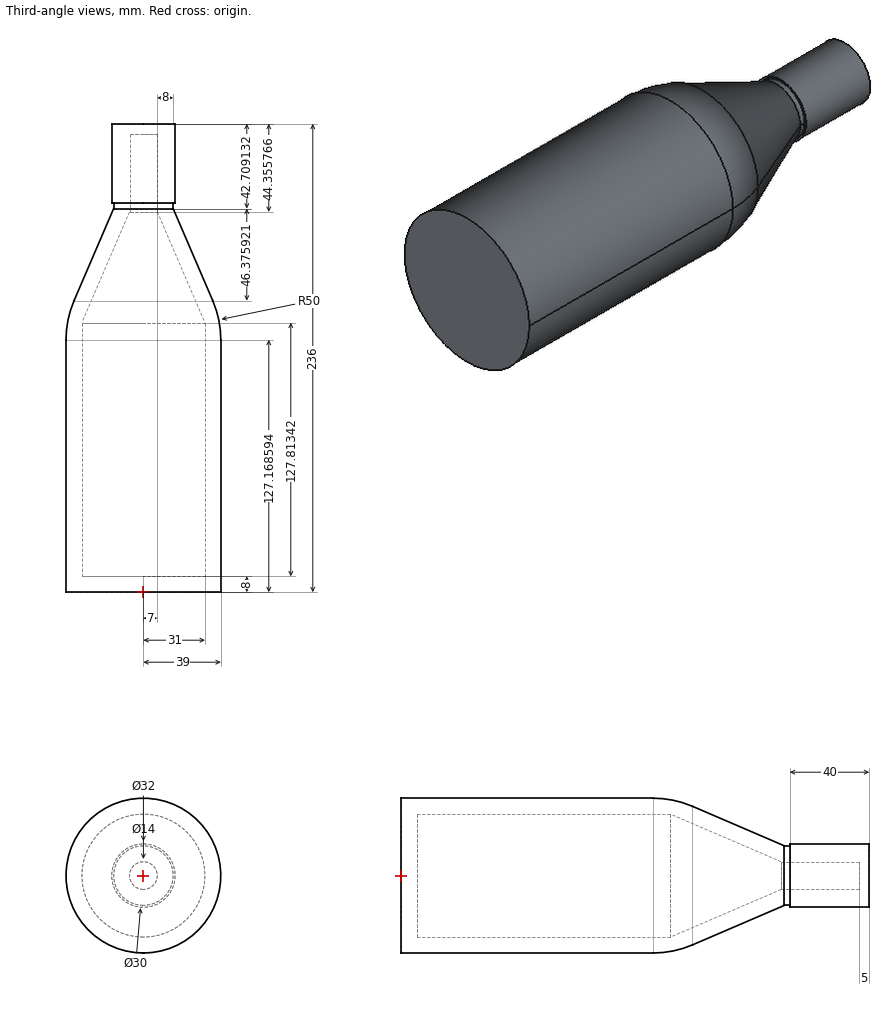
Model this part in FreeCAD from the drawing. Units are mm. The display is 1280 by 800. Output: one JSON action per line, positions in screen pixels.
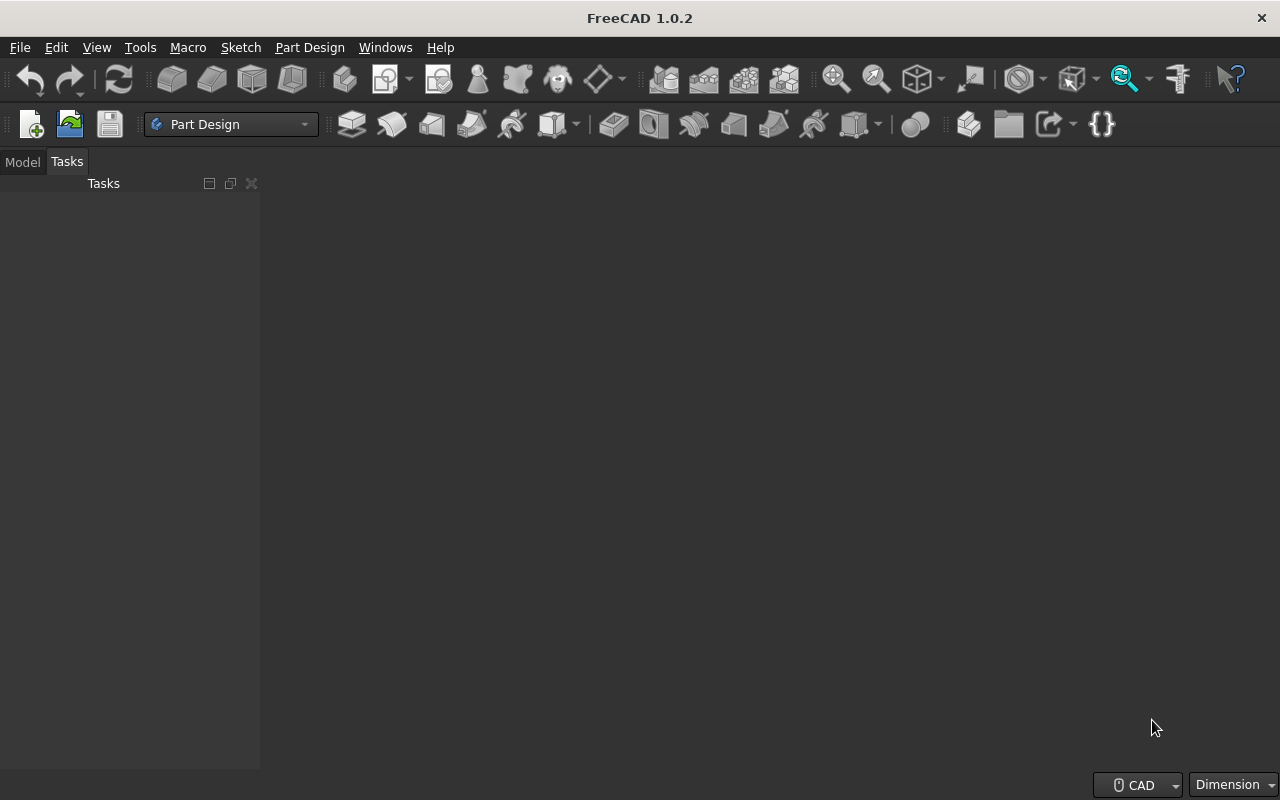
{"action": "key", "text": "ctrl+n"}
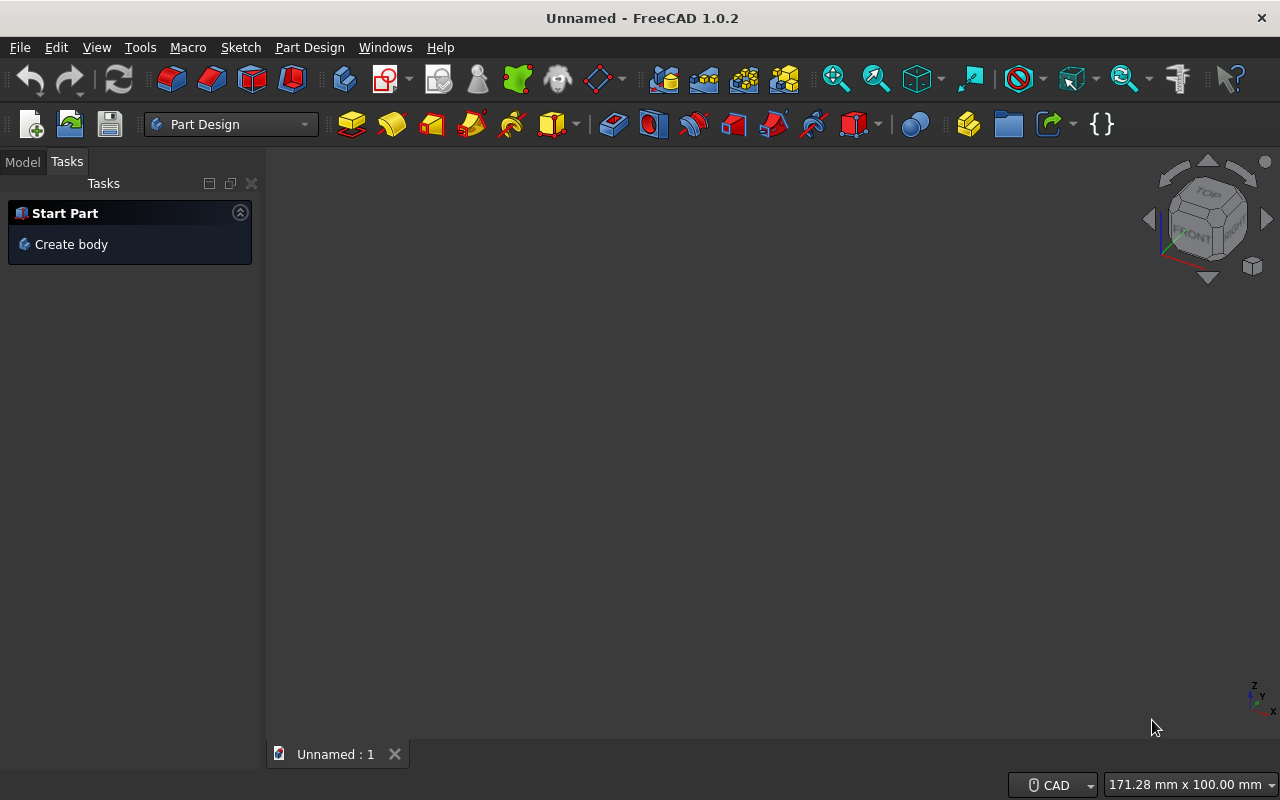
{"action": "left_click", "coordinate": [386, 80]}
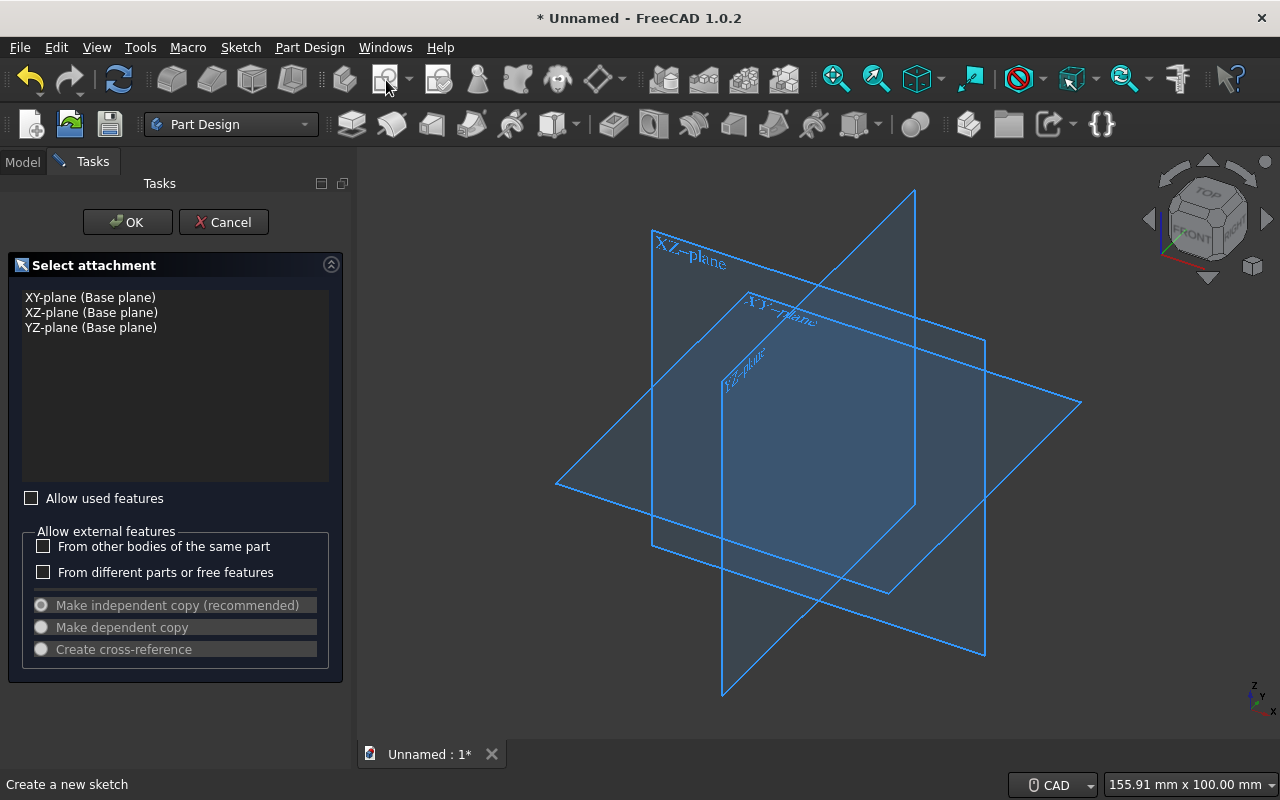
{"action": "left_click", "coordinate": [82, 298]}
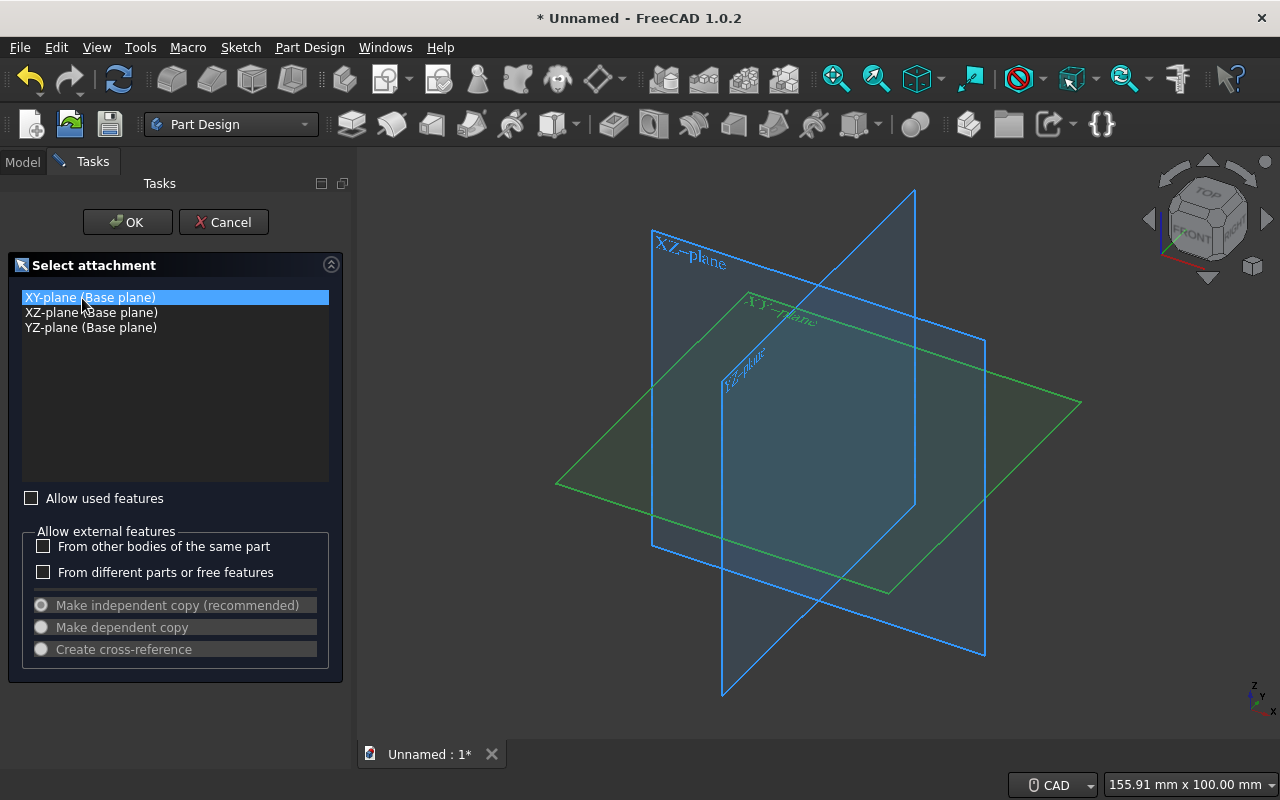
{"action": "left_click", "coordinate": [128, 222]}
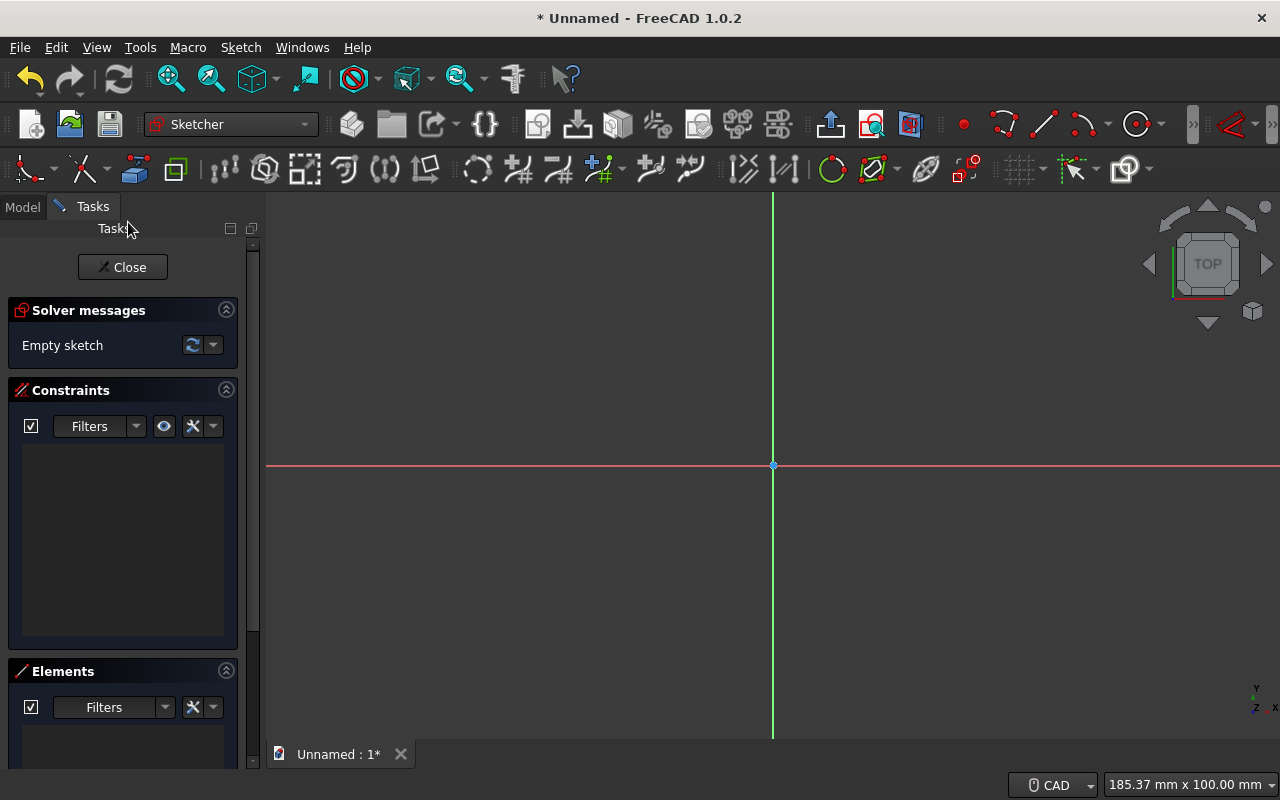
{"action": "scroll", "coordinate": [647, 677], "scroll_direction": "down", "scroll_amount": 7}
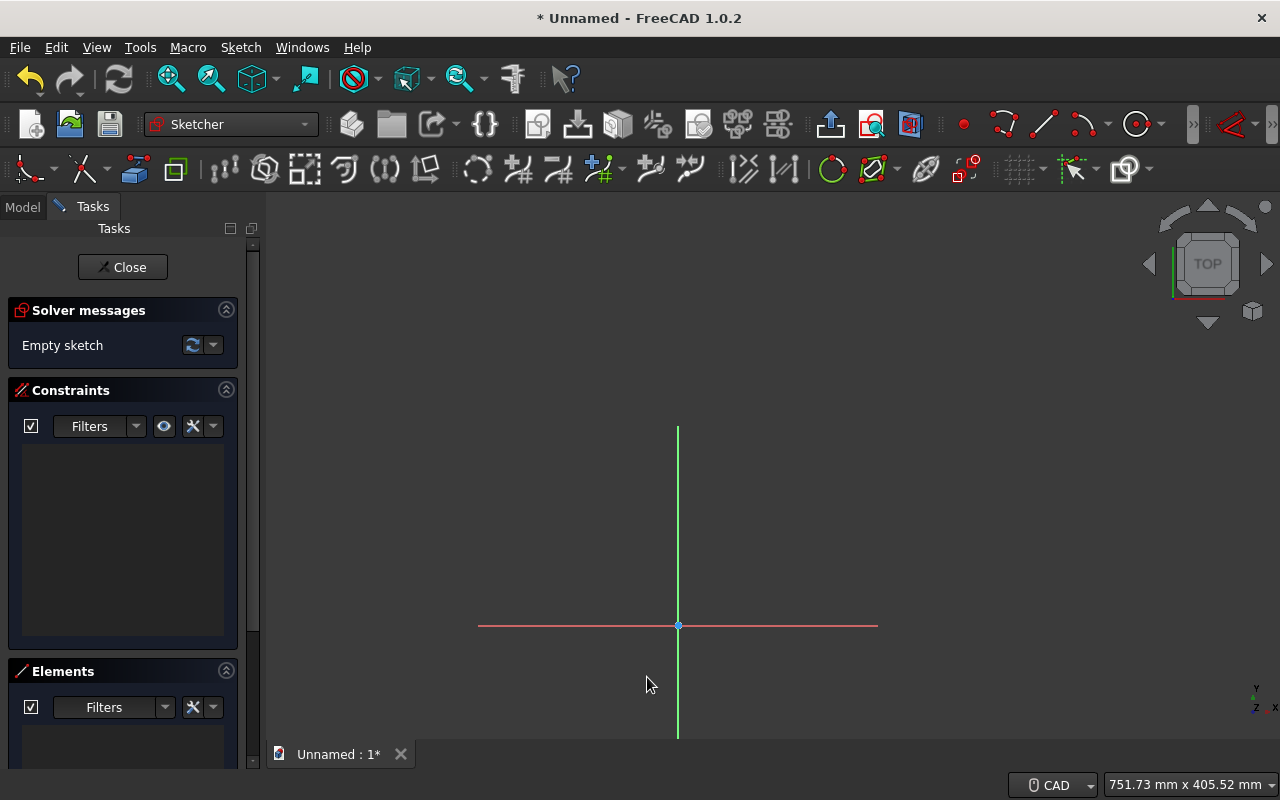
{"action": "left_click", "coordinate": [1004, 124]}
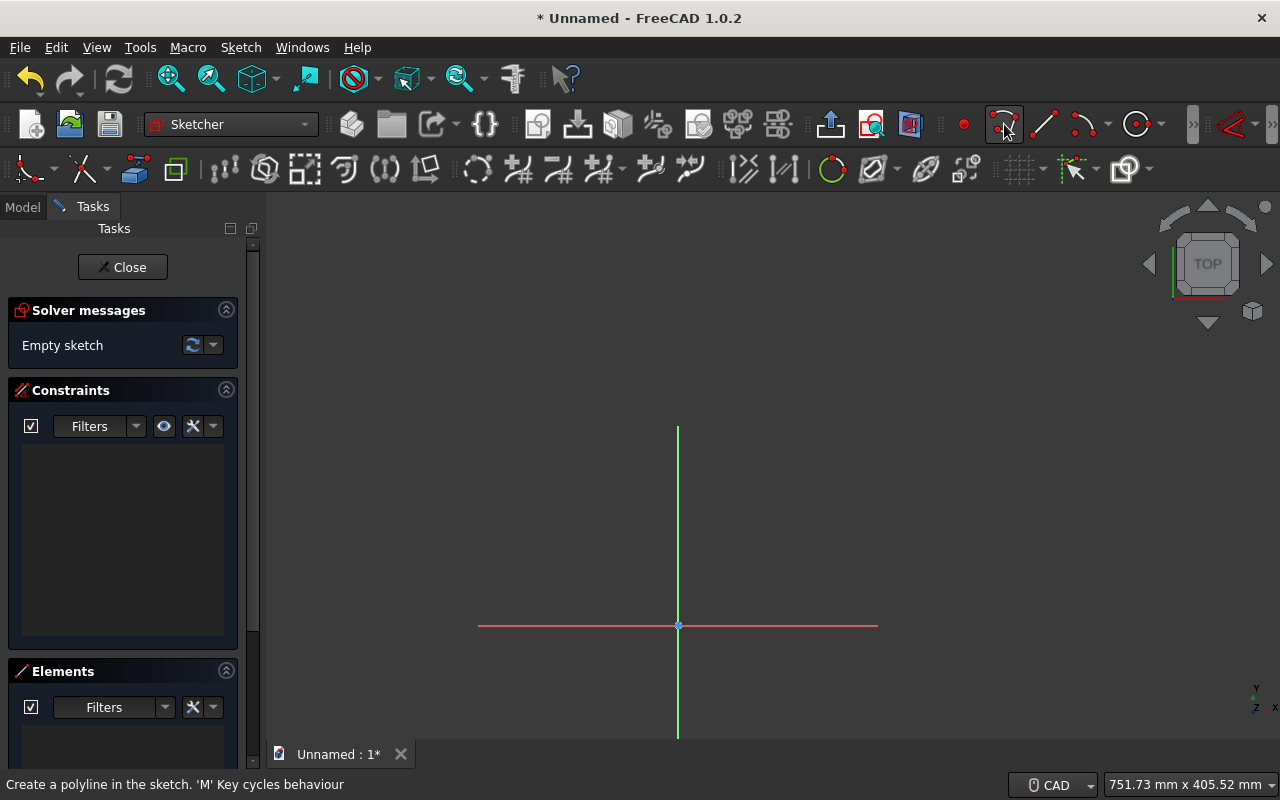
{"action": "left_click", "coordinate": [725, 427]}
{"action": "left_click", "coordinate": [699, 365]}
{"action": "left_click", "coordinate": [699, 307]}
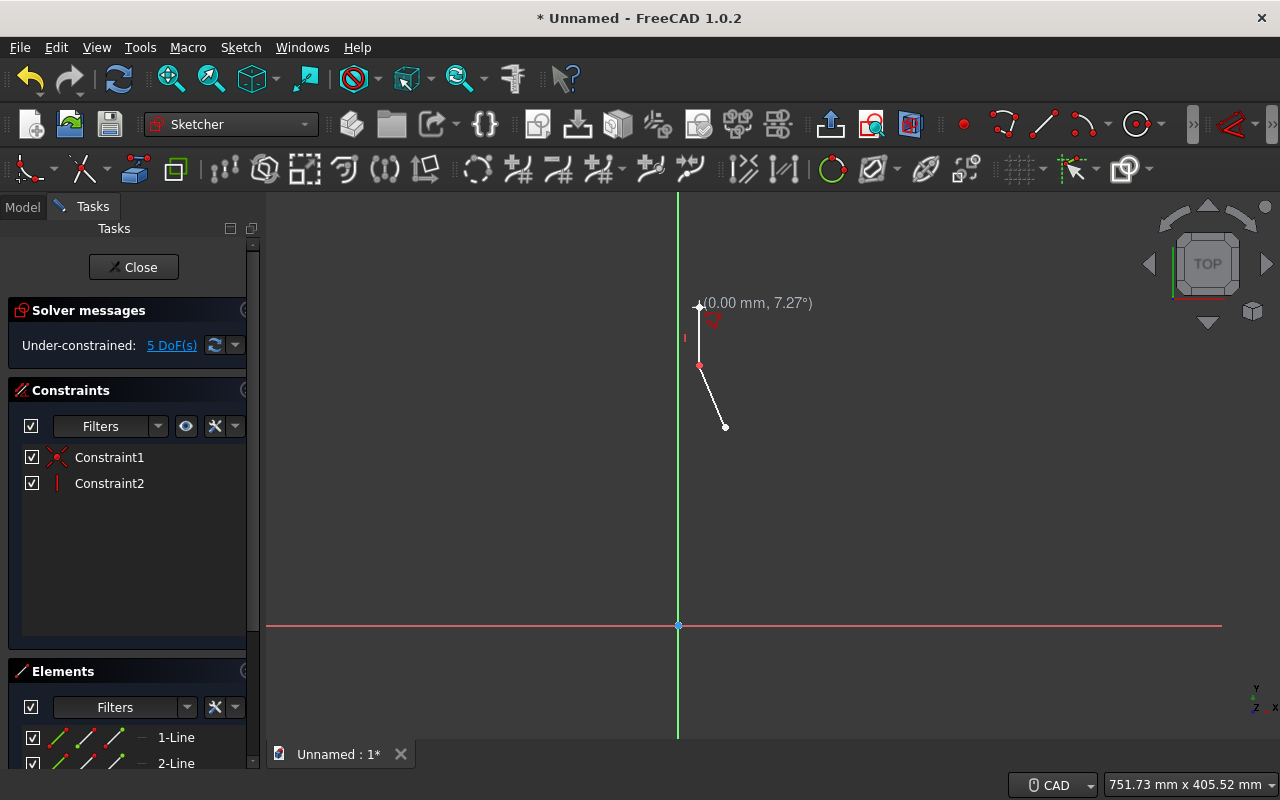
{"action": "scroll", "coordinate": [688, 307], "scroll_direction": "up", "scroll_amount": 3}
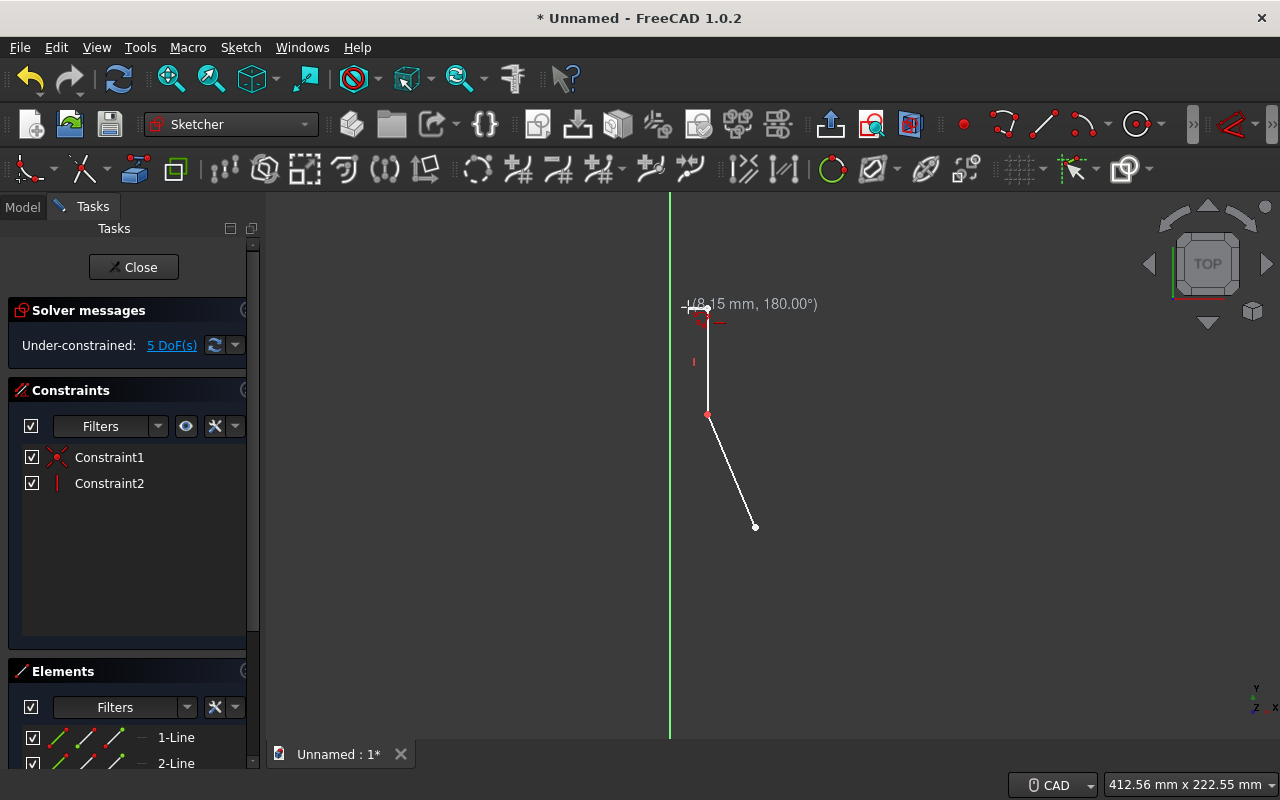
{"action": "left_click", "coordinate": [687, 307]}
{"action": "left_click", "coordinate": [687, 416]}
{"action": "left_click", "coordinate": [746, 553]}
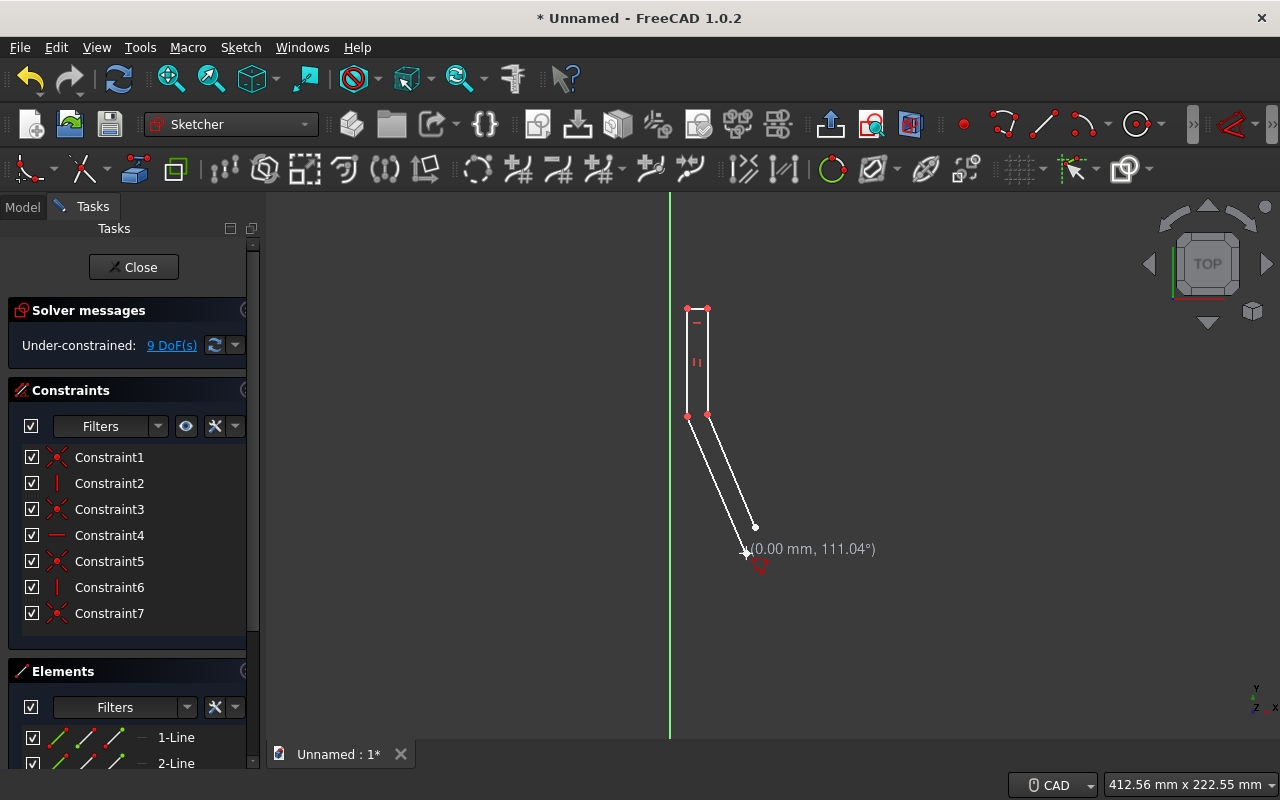
{"action": "scroll", "coordinate": [688, 305], "scroll_direction": "down", "scroll_amount": 3}